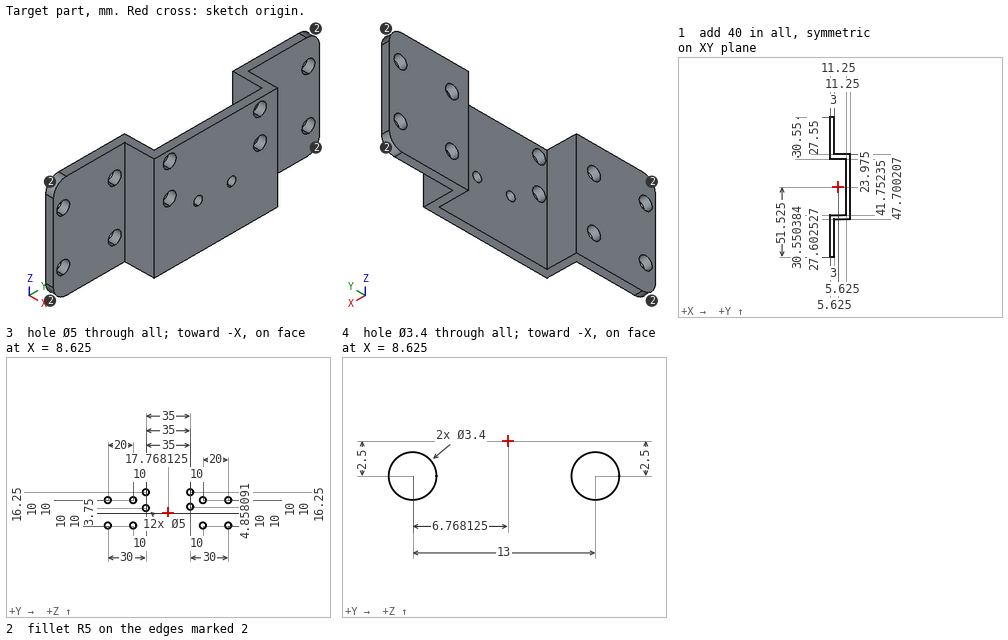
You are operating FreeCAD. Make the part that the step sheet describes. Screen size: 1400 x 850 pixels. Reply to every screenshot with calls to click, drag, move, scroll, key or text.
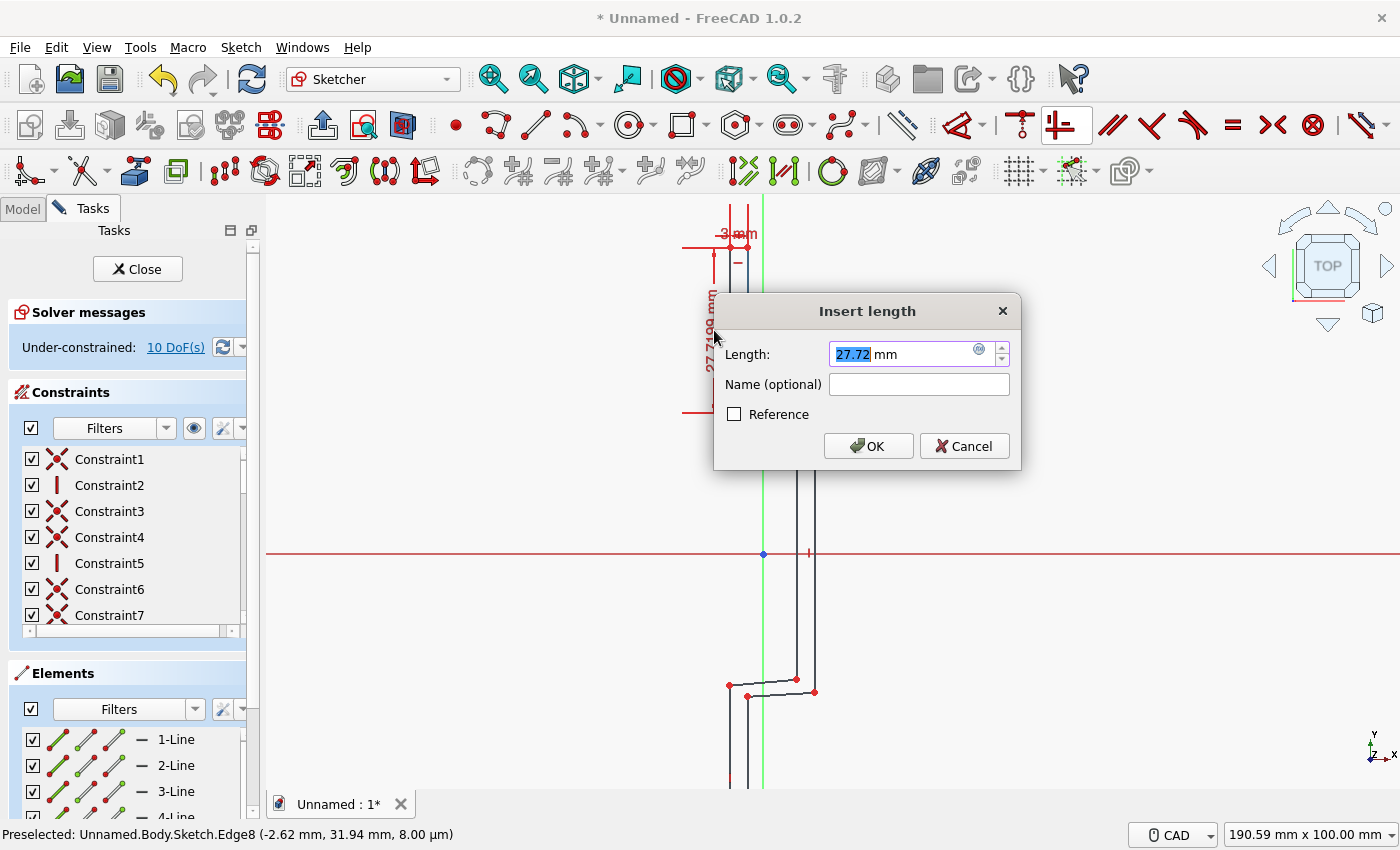
text(27.55)
key(Return)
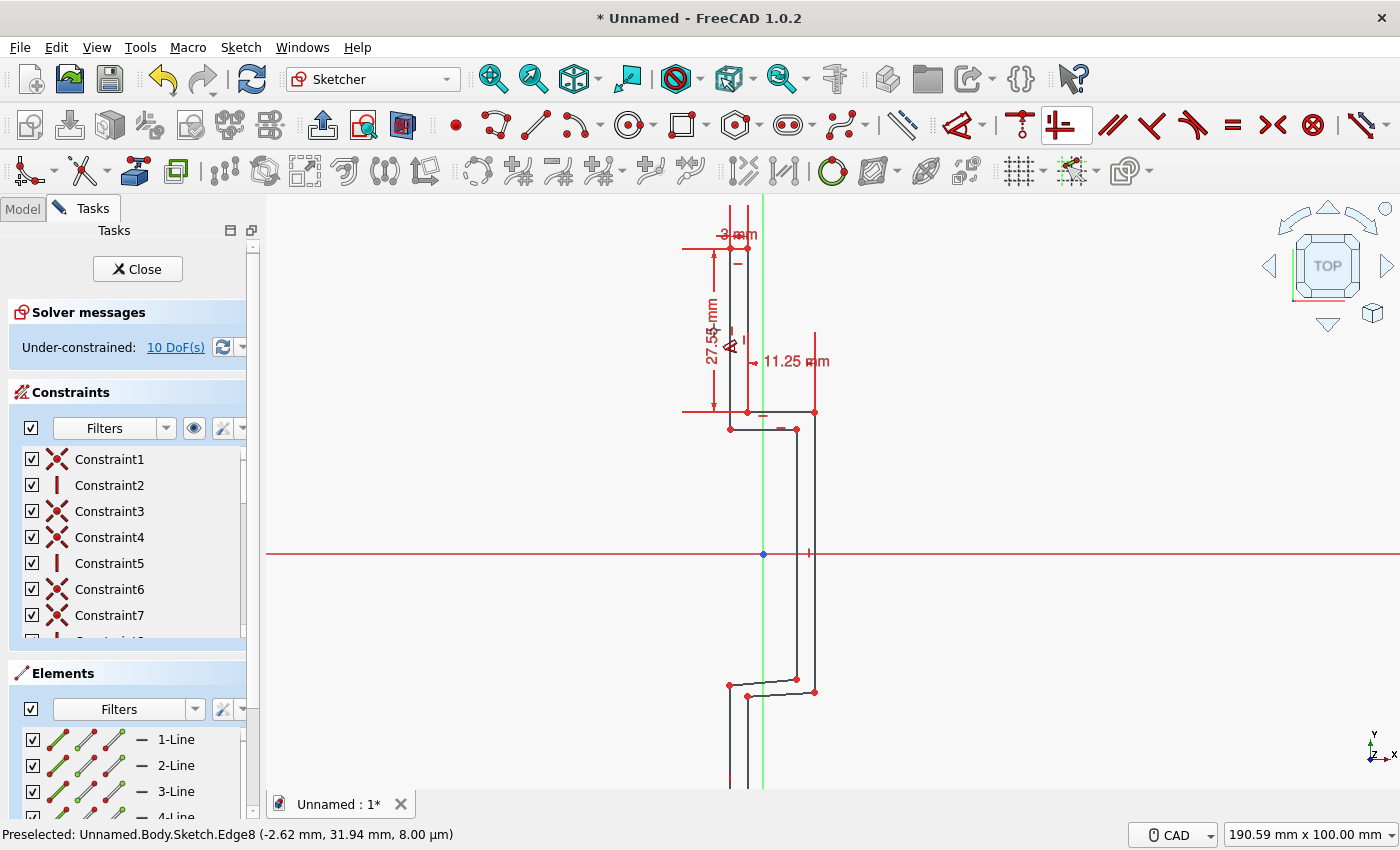
click(730, 303)
click(696, 298)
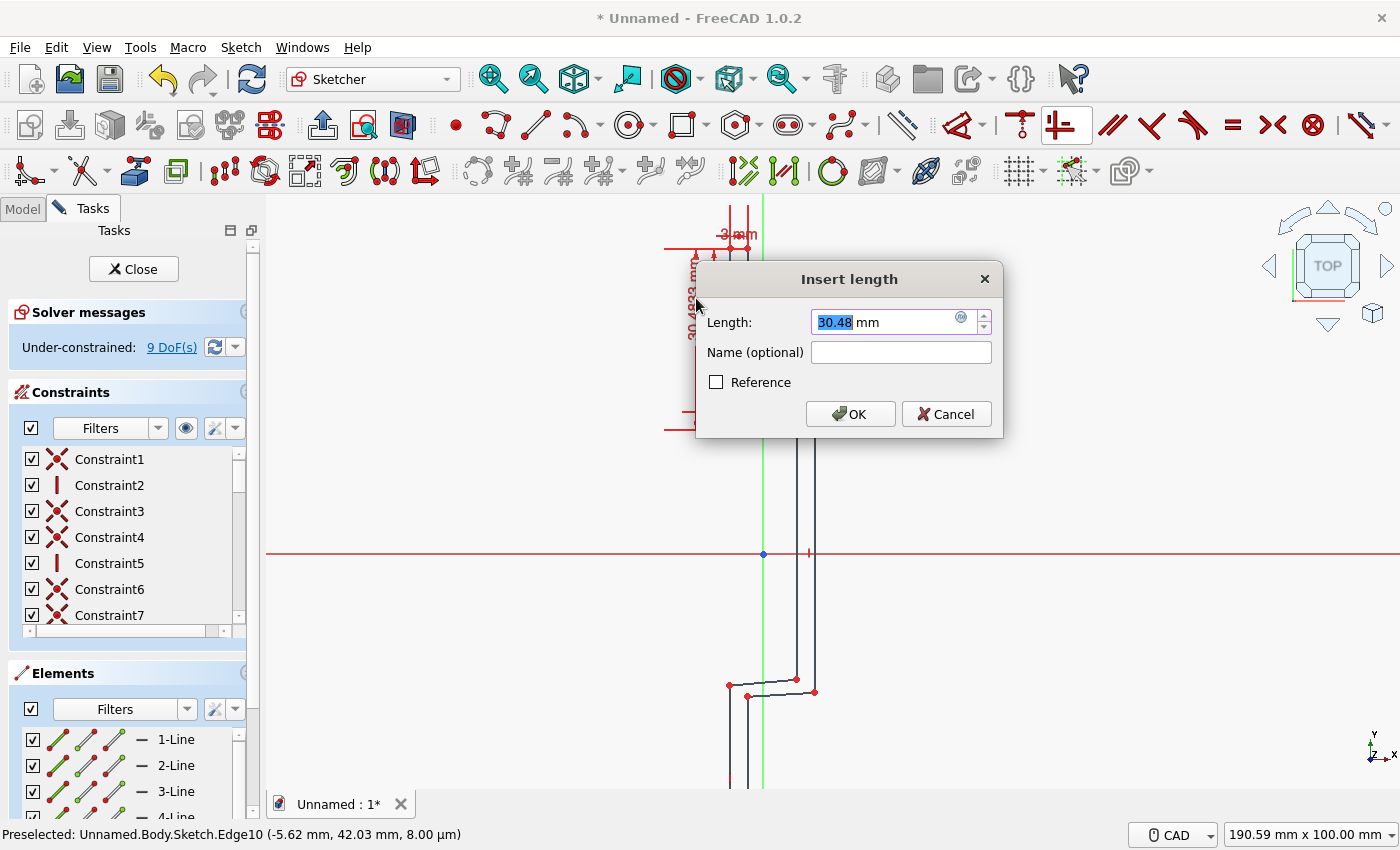
text(30.55)
key(Return)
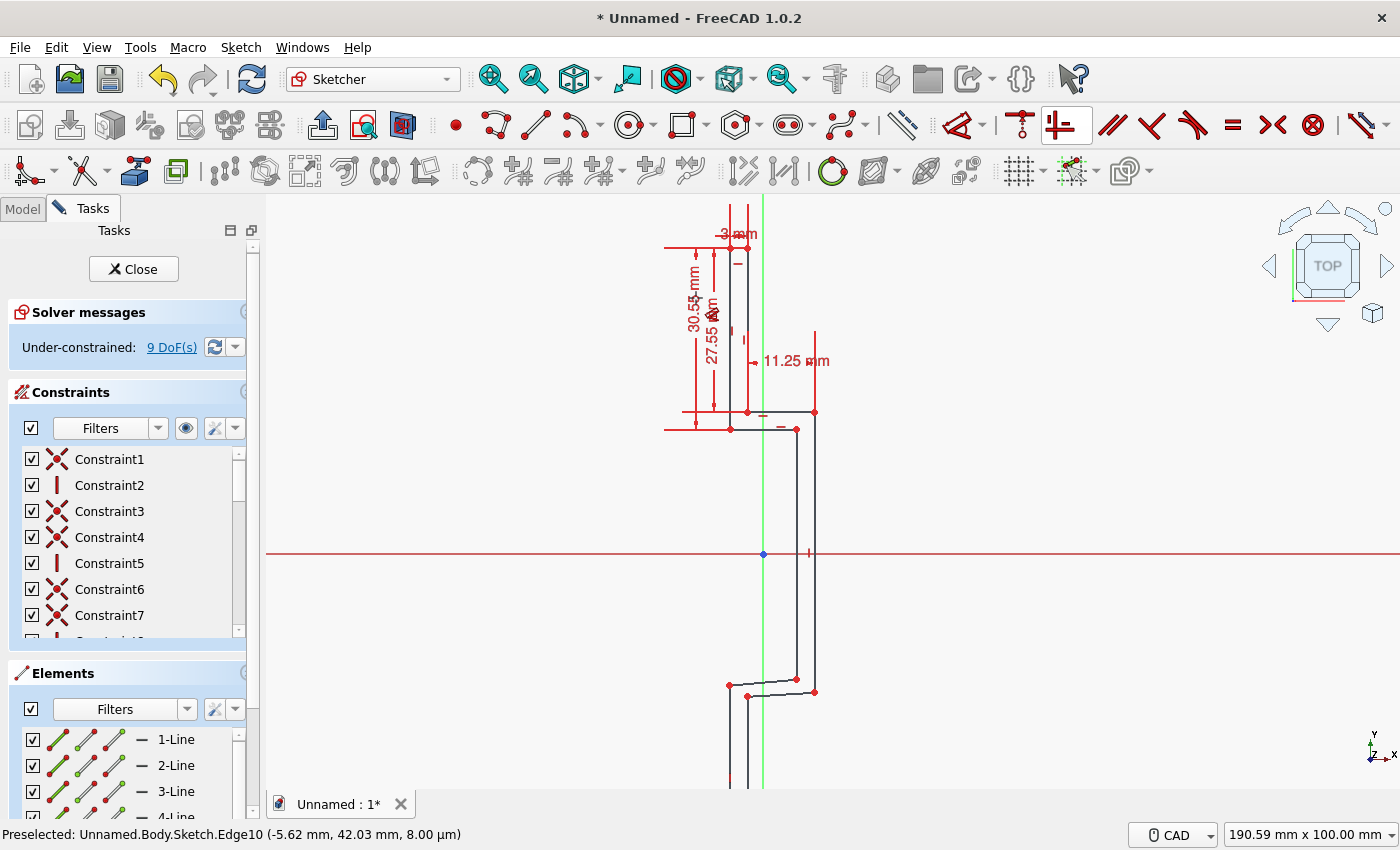
click(750, 430)
click(779, 396)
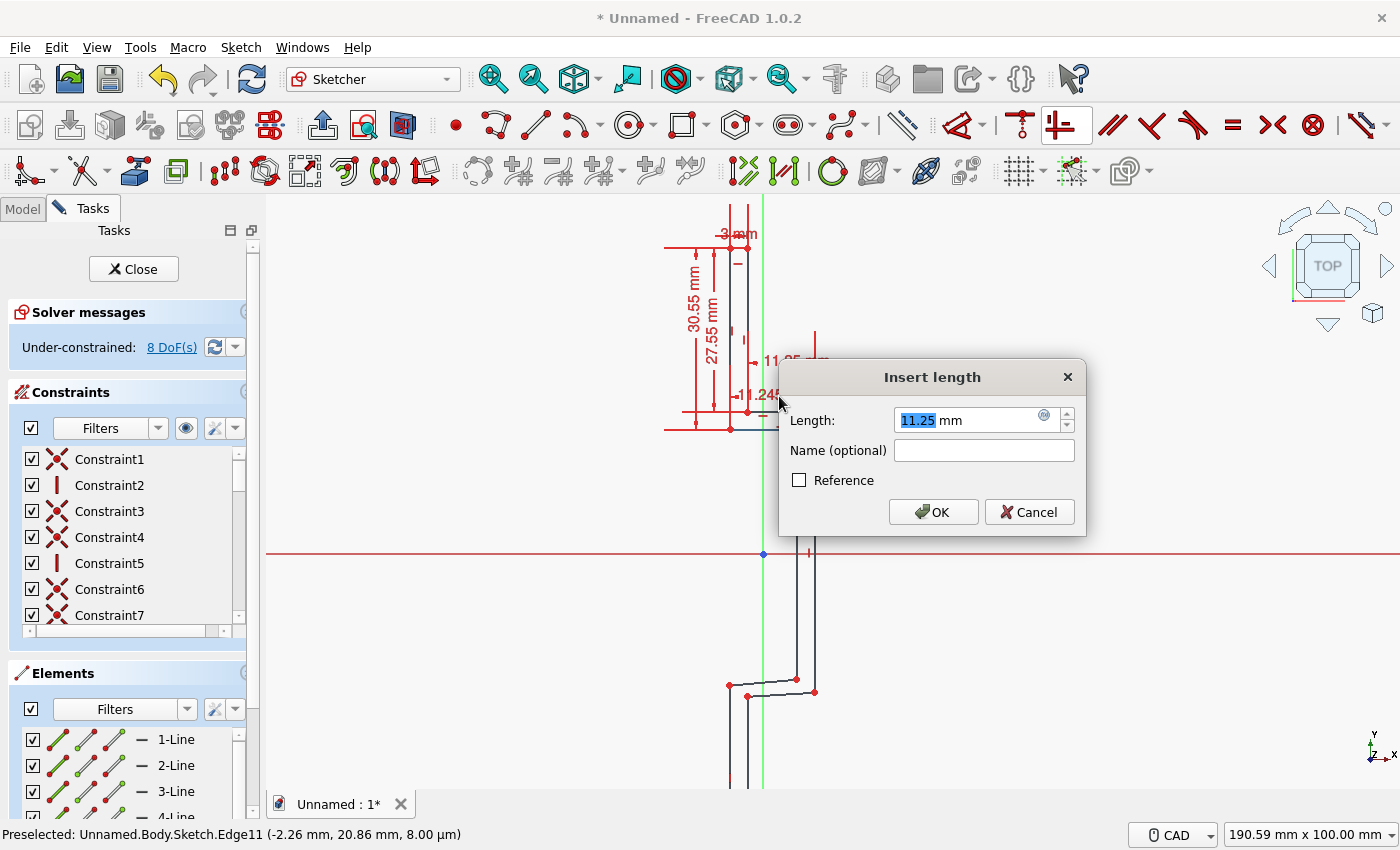
text(11.25)
key(Return)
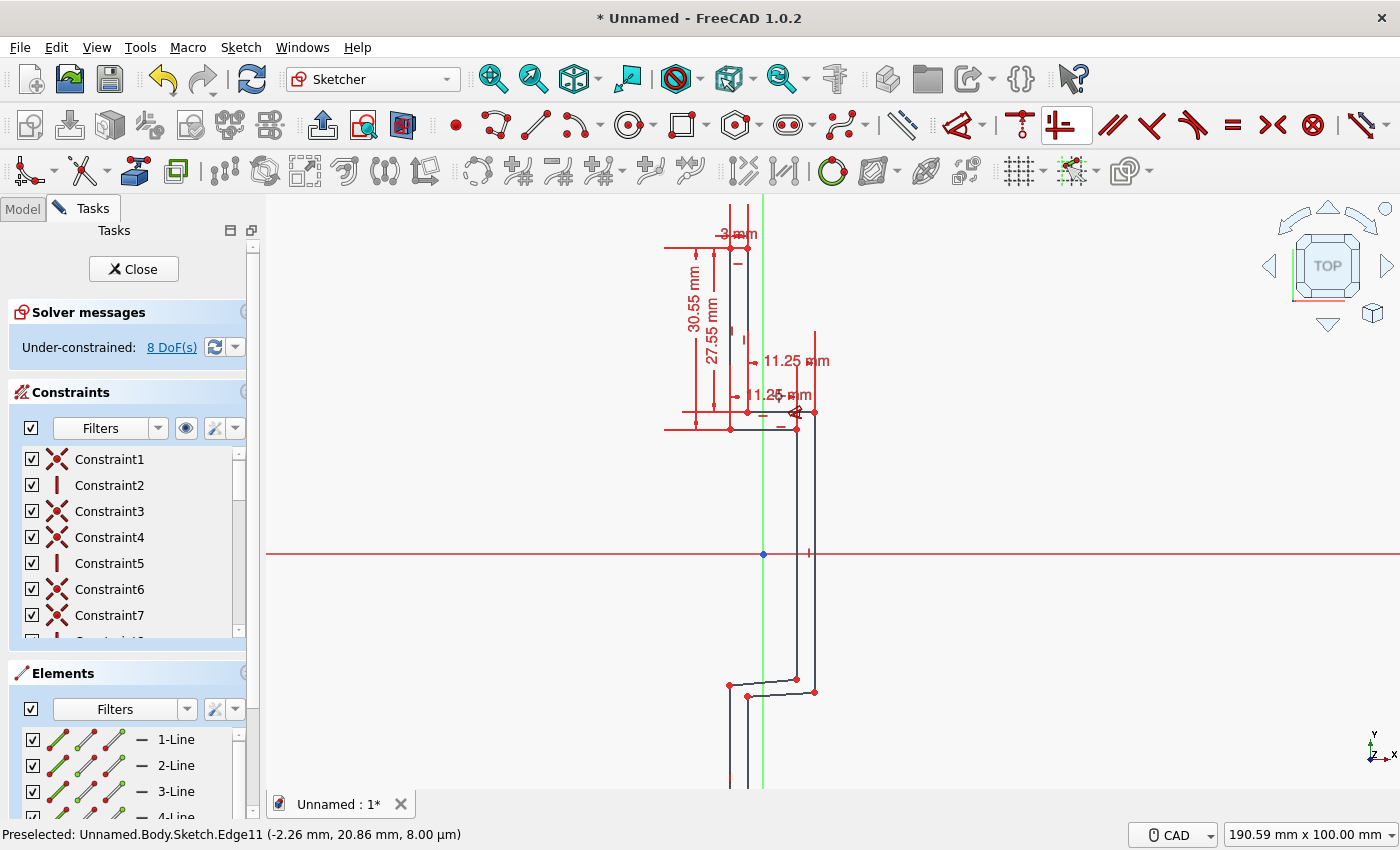
click(797, 680)
click(780, 714)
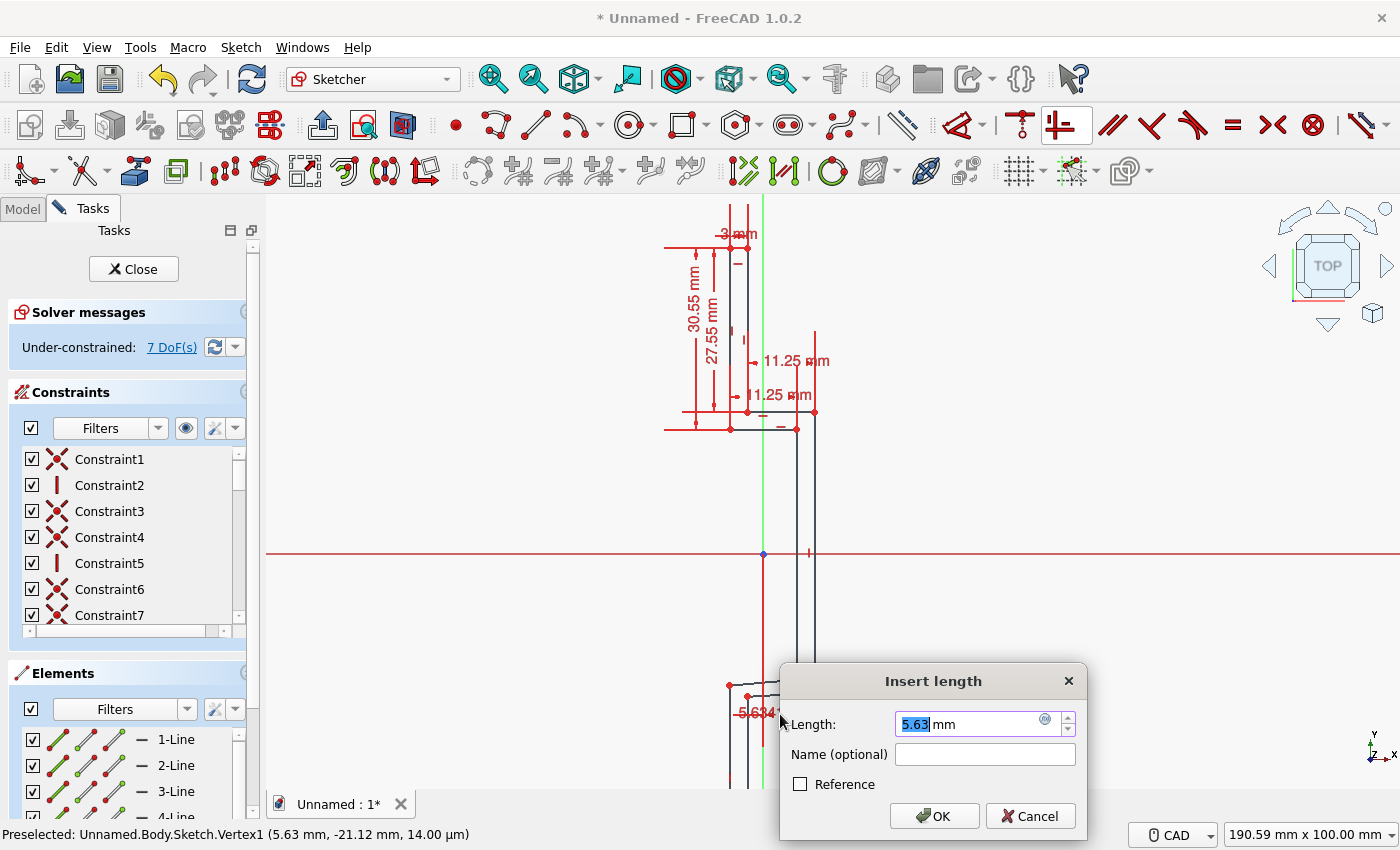
text(5.625)
key(Return)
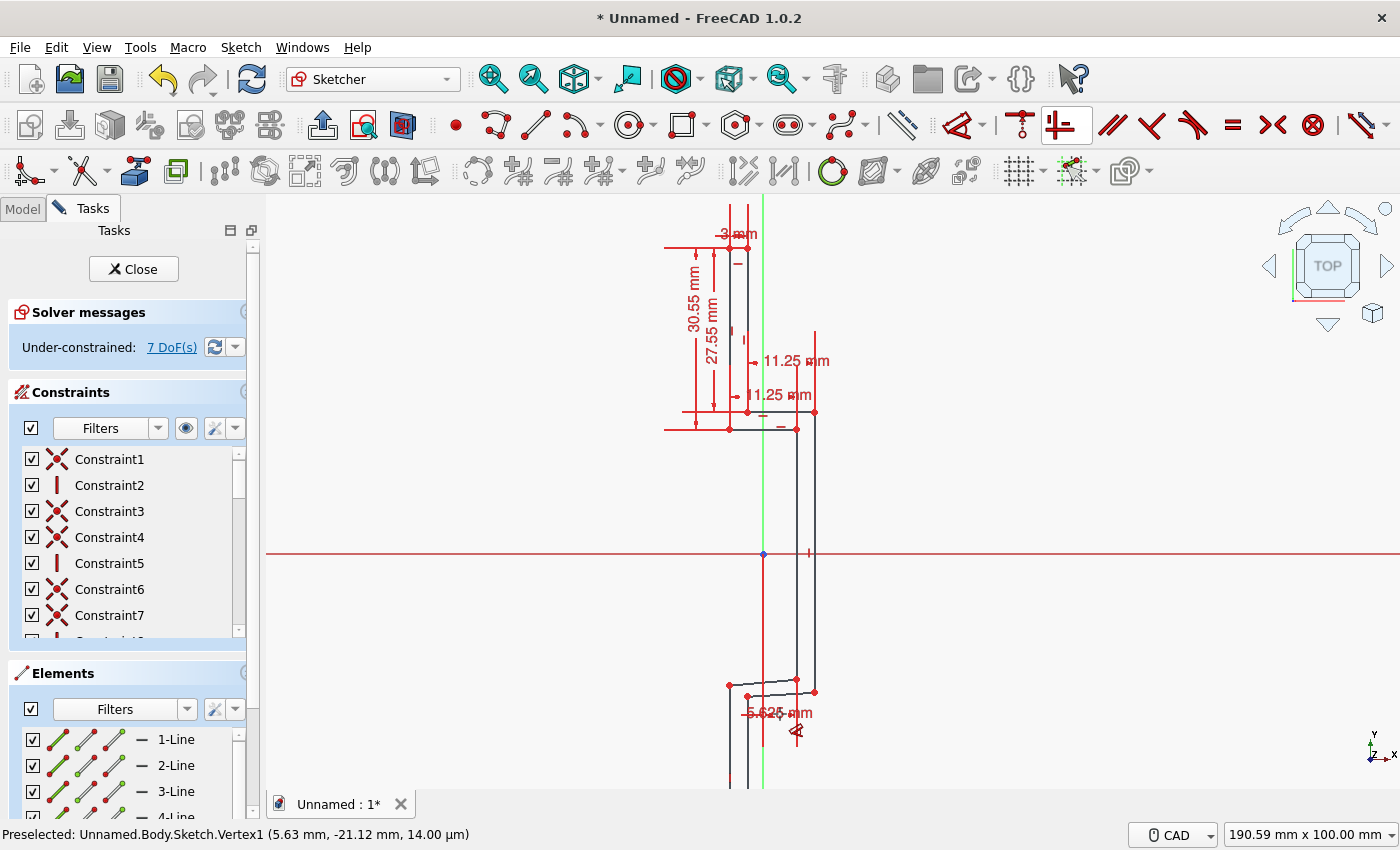
click(730, 686)
click(747, 520)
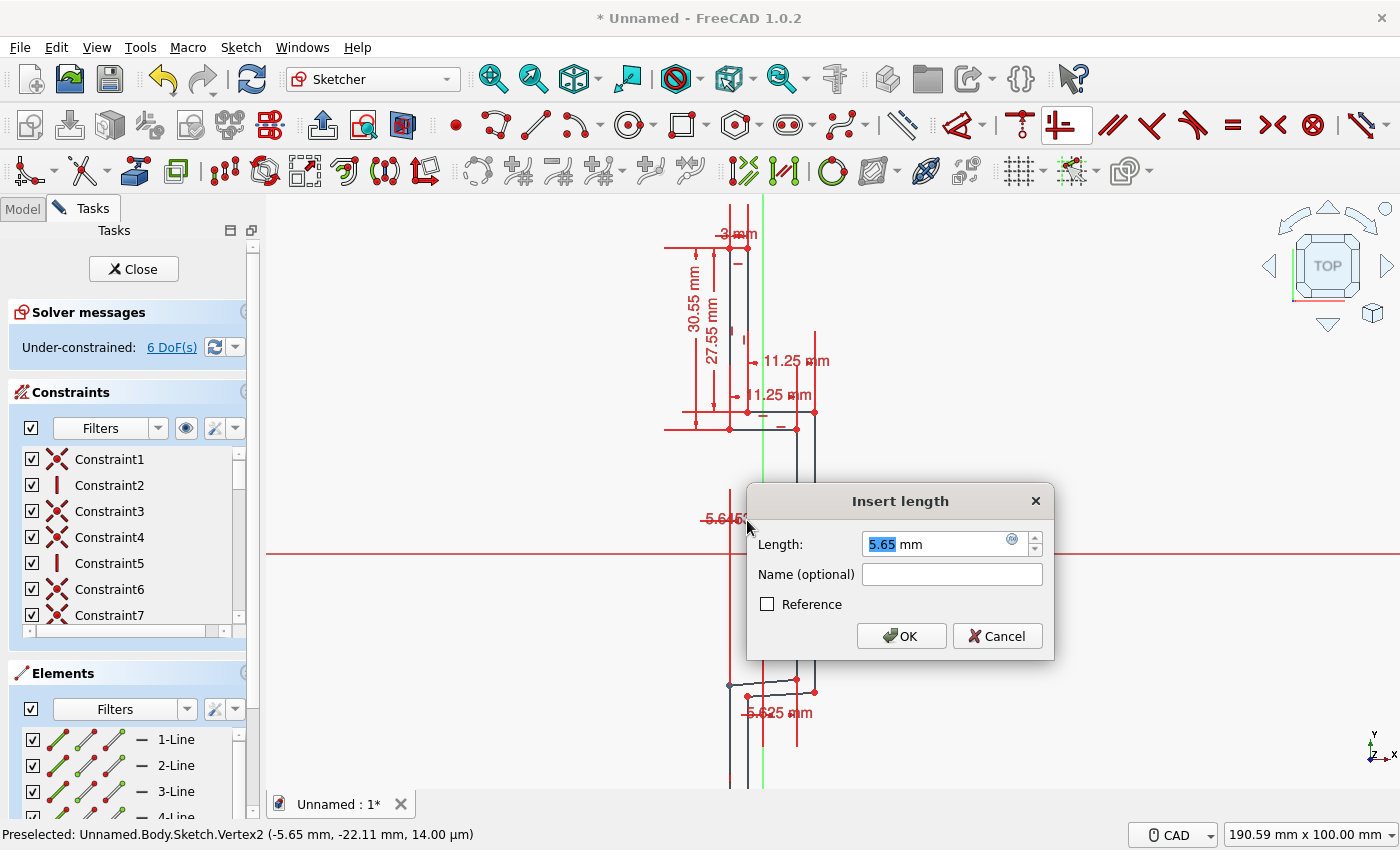
text(5.625)
key(Return)